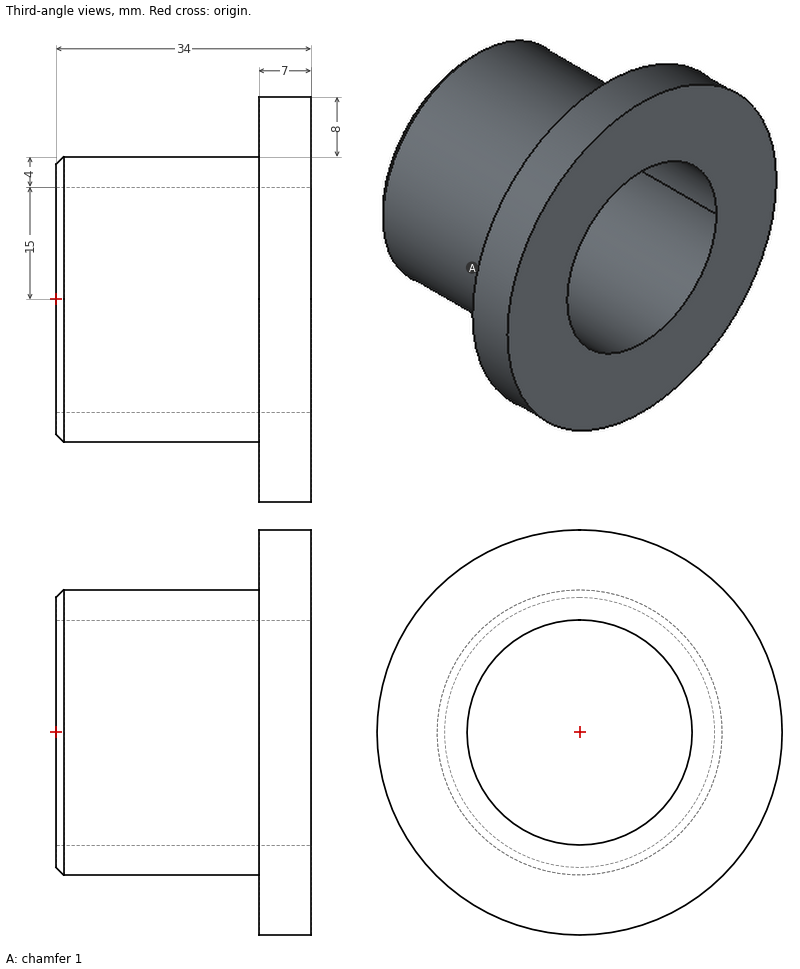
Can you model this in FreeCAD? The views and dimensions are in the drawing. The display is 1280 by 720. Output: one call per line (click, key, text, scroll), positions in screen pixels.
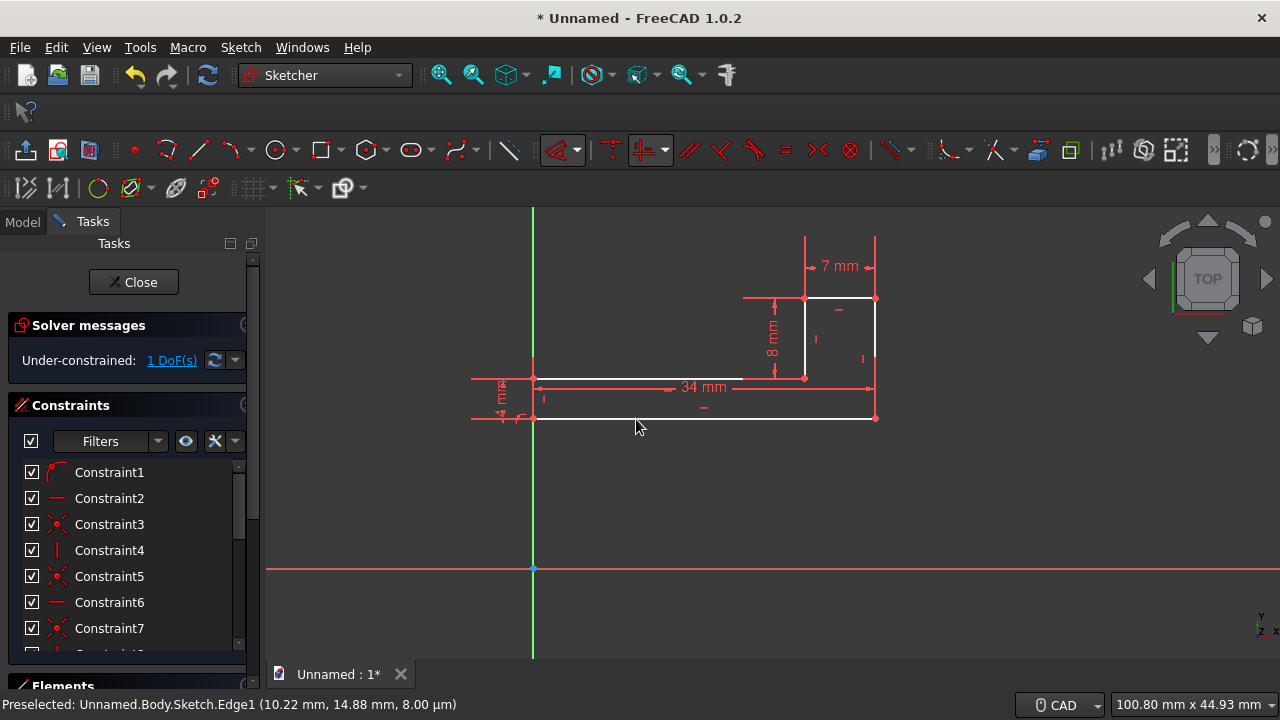
click(533, 419)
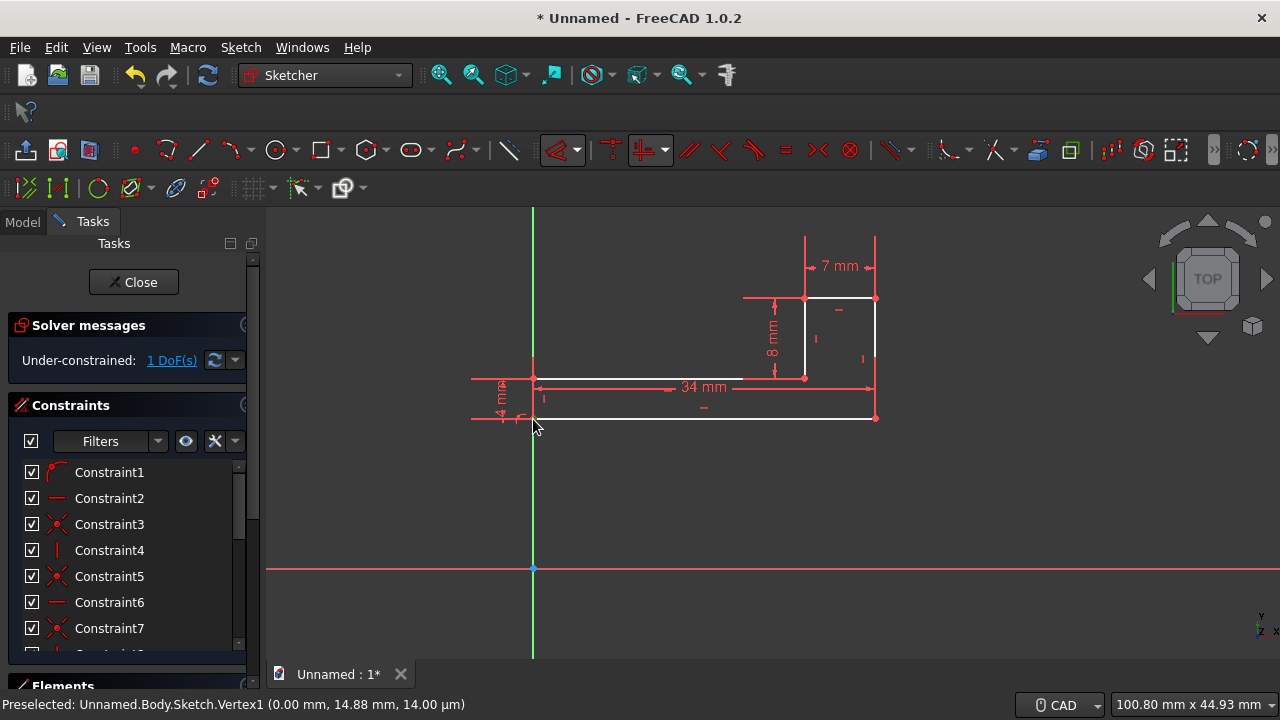
key(i)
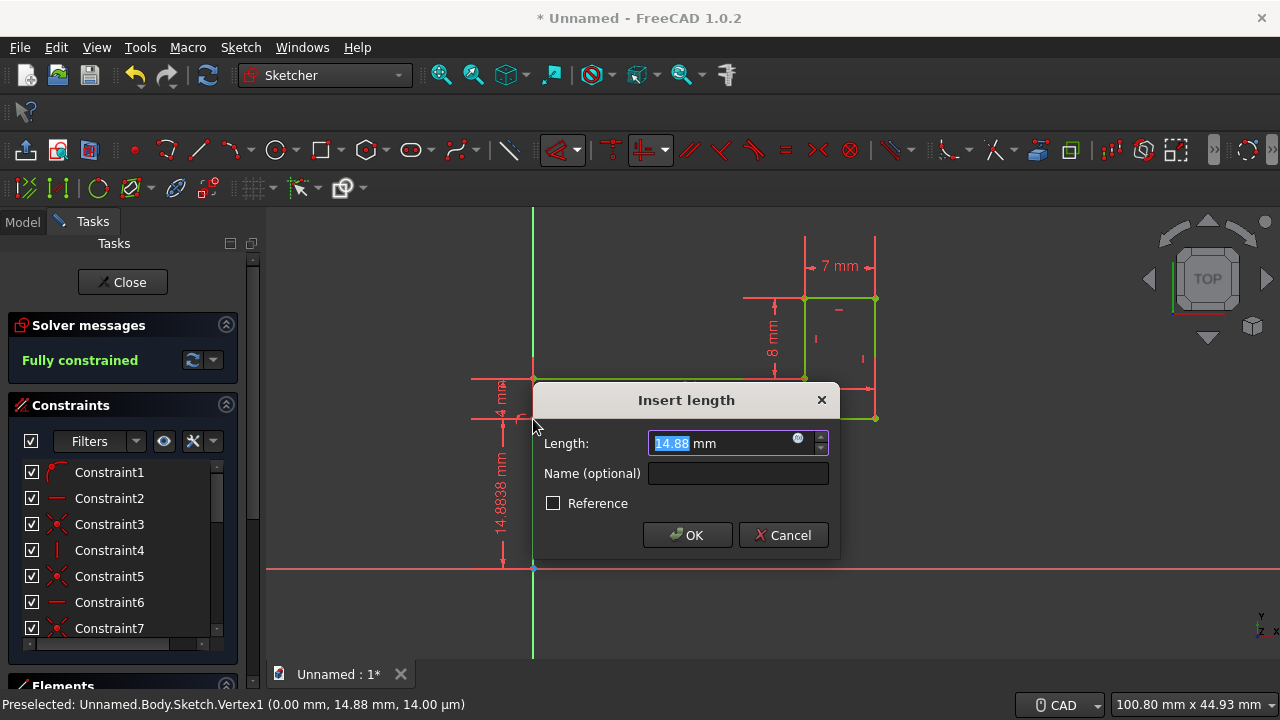
text(15)
key(Return)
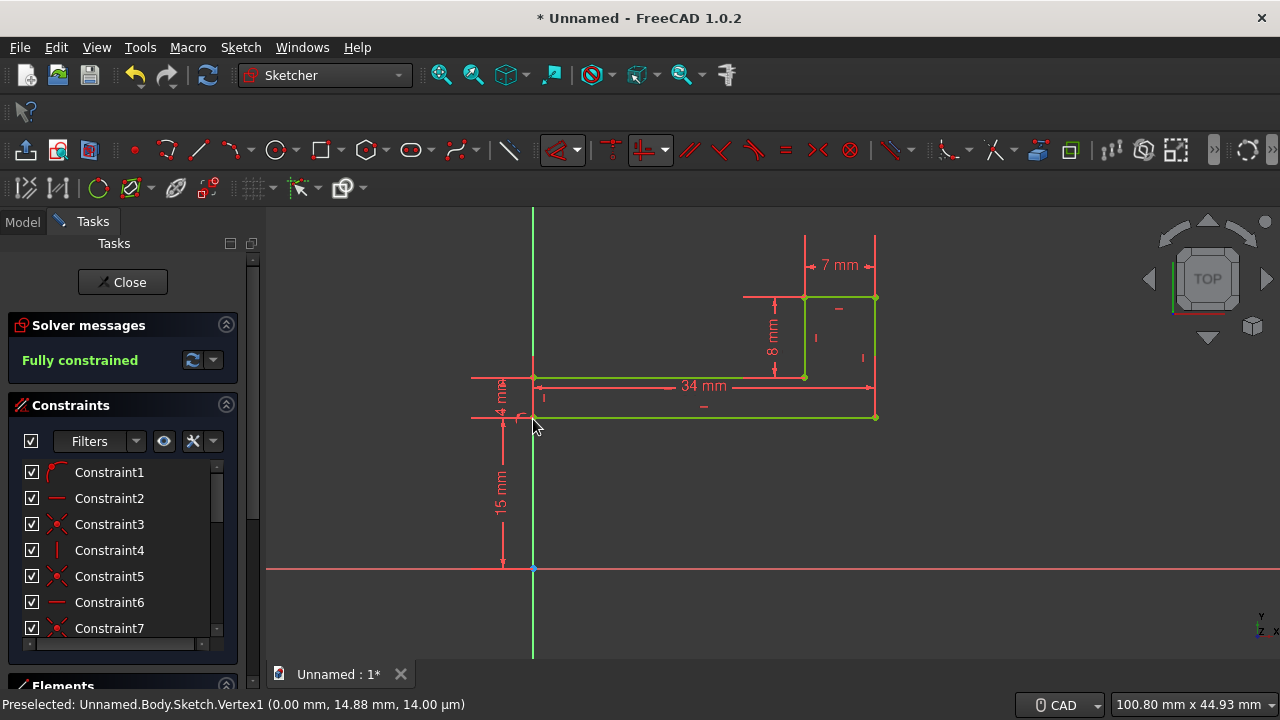
click(123, 282)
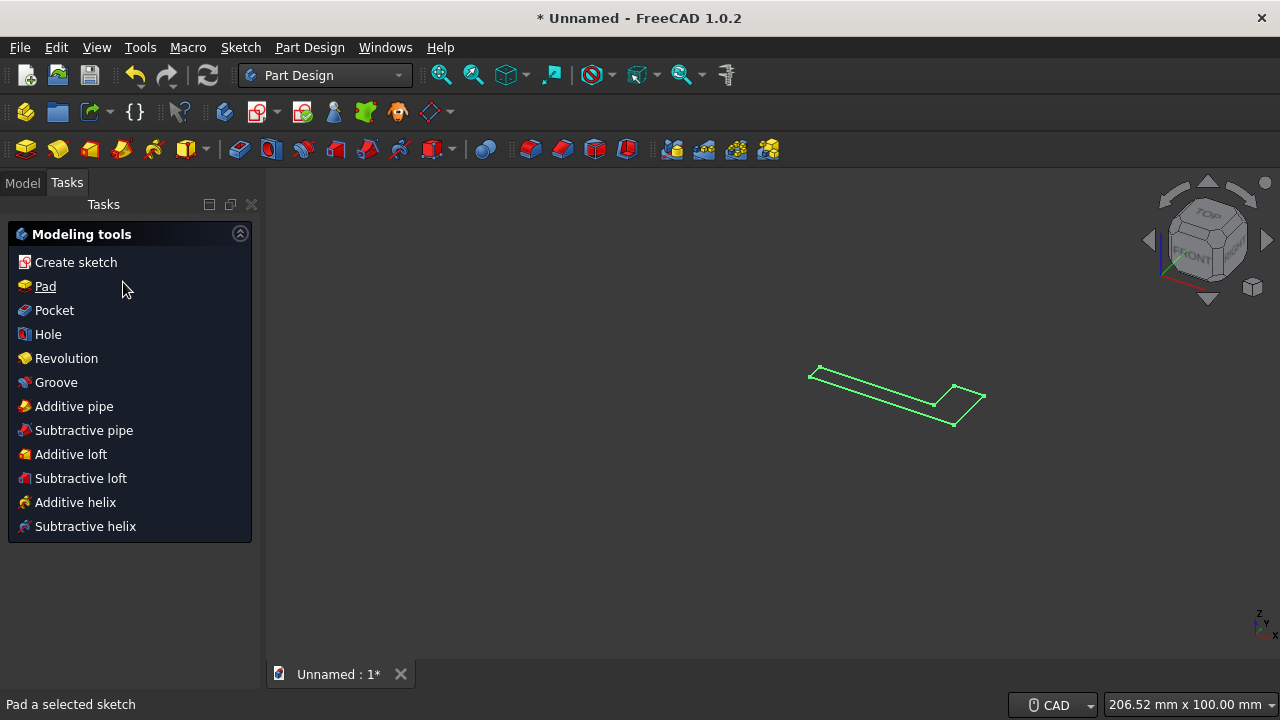
click(58, 150)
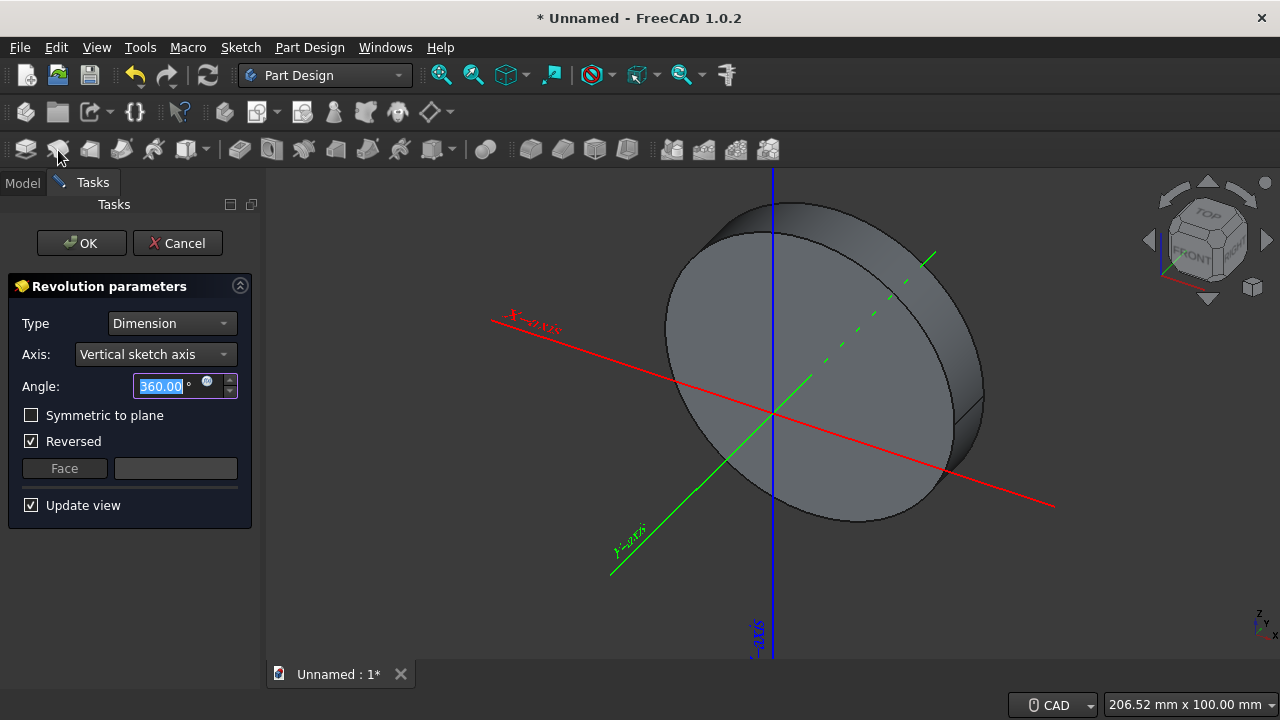
click(156, 354)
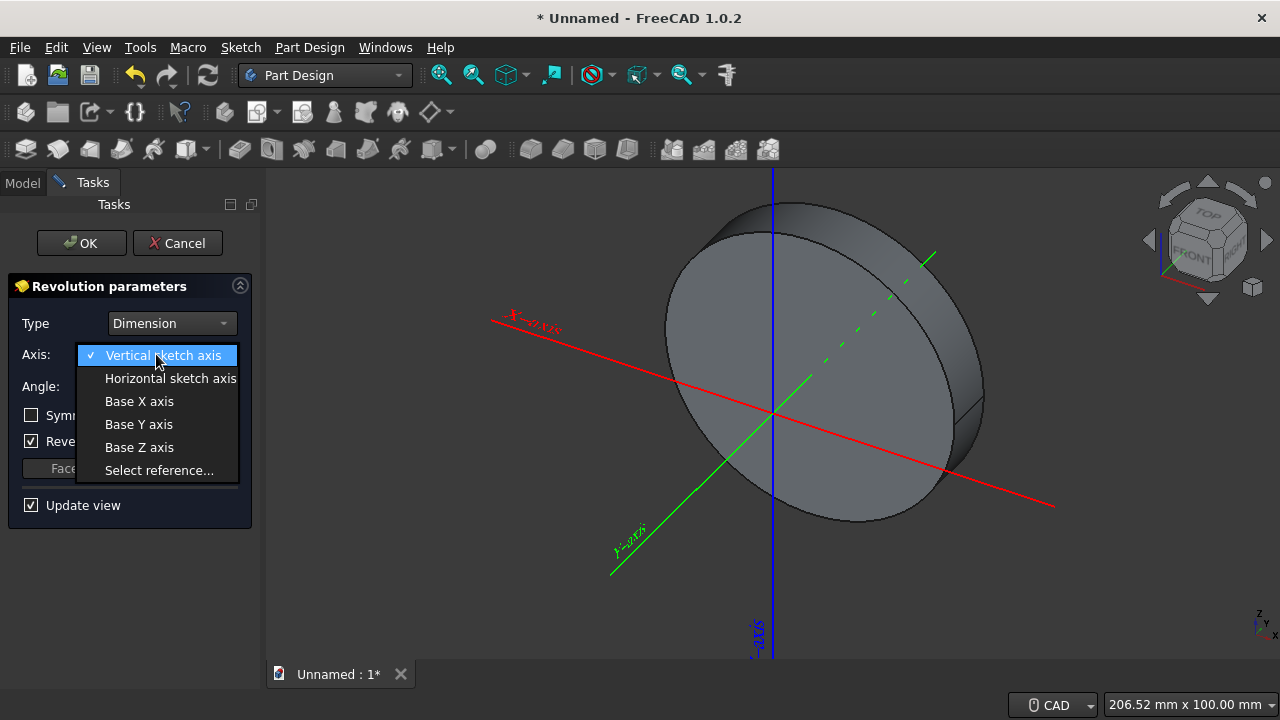
click(156, 378)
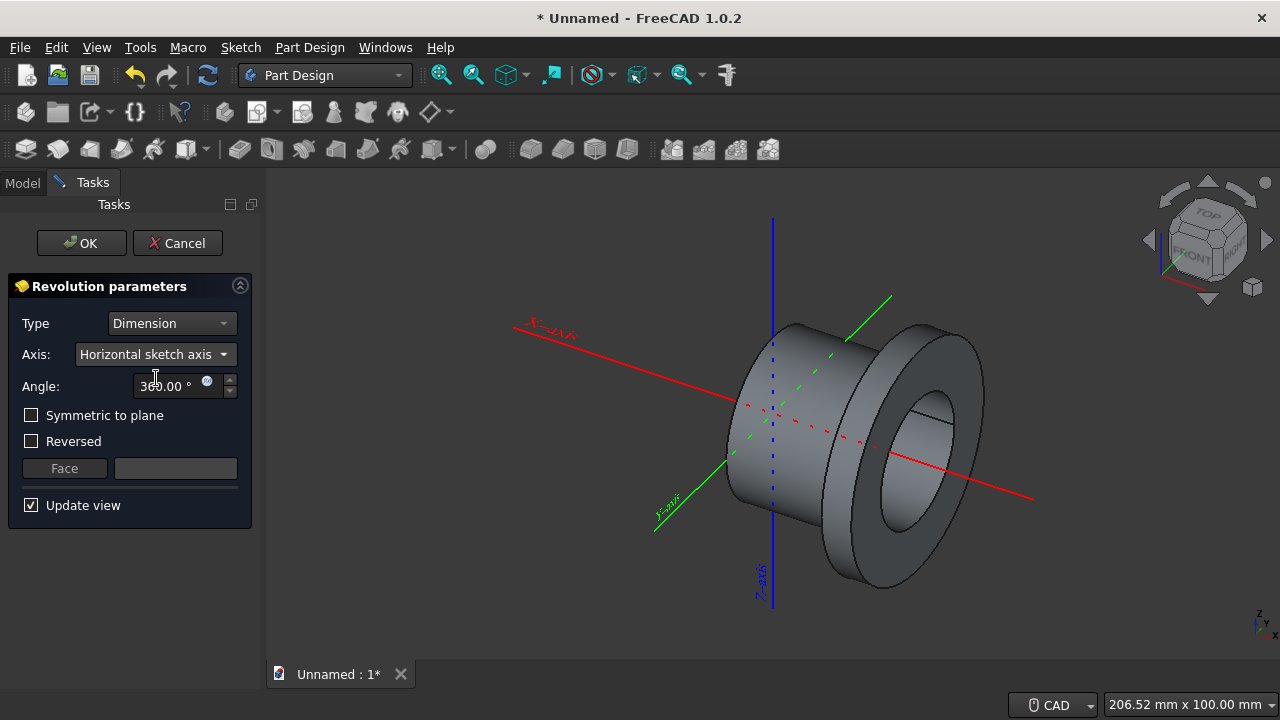
click(82, 243)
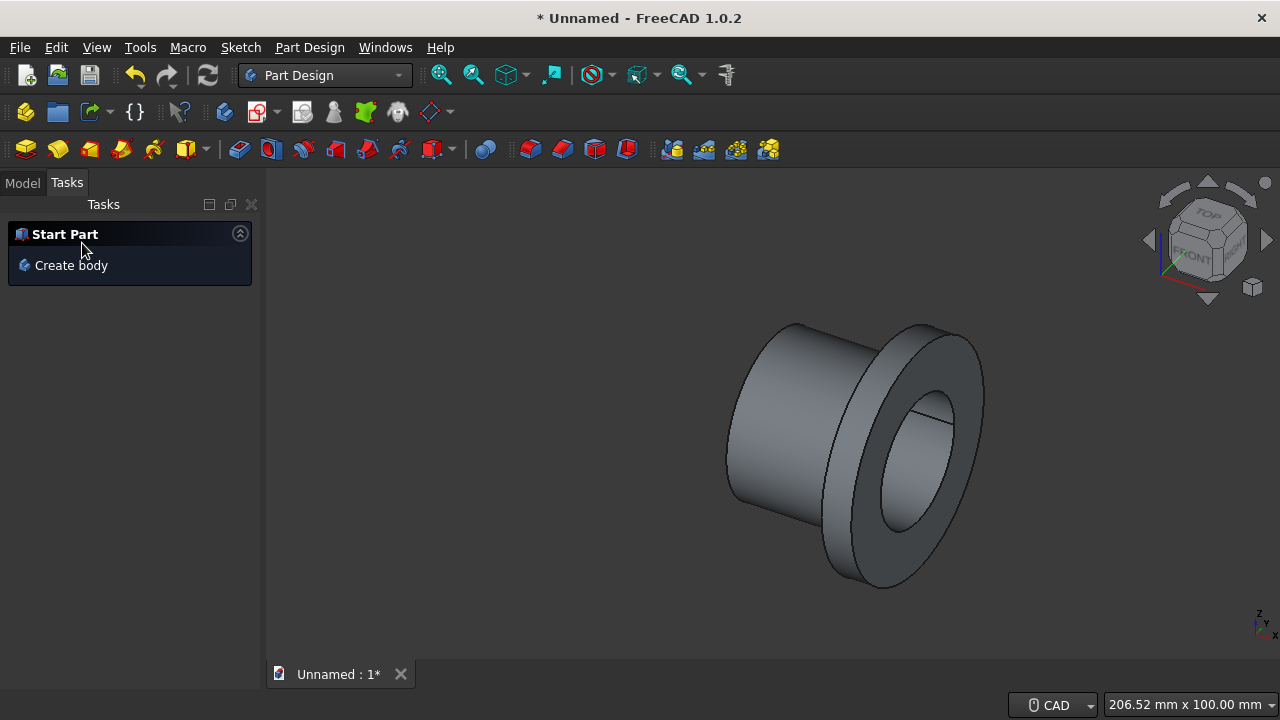
key(0)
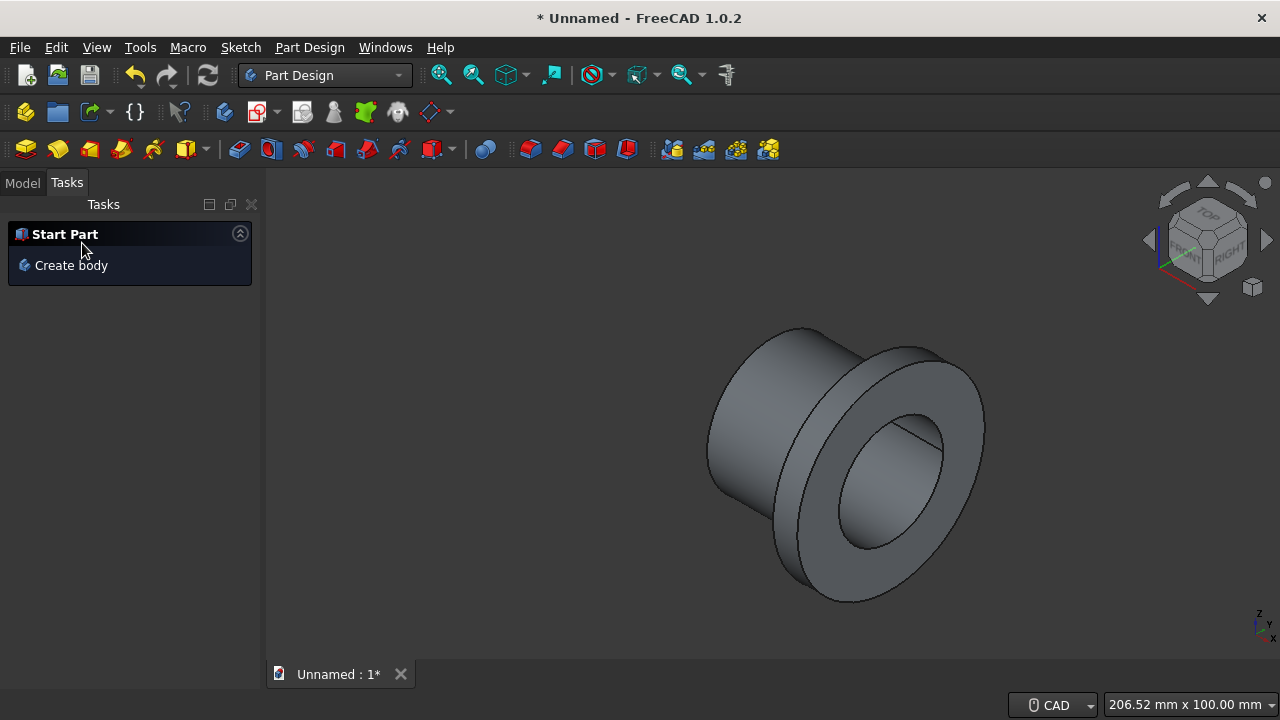
key(2)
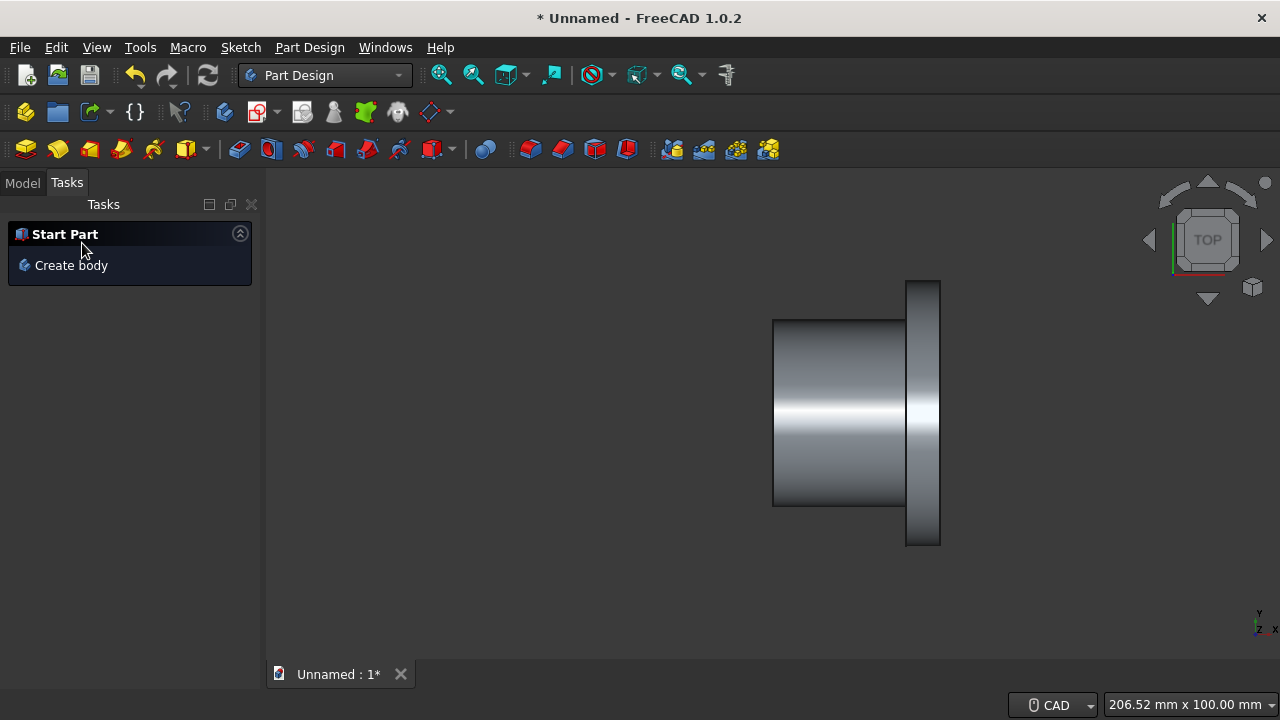
click(773, 488)